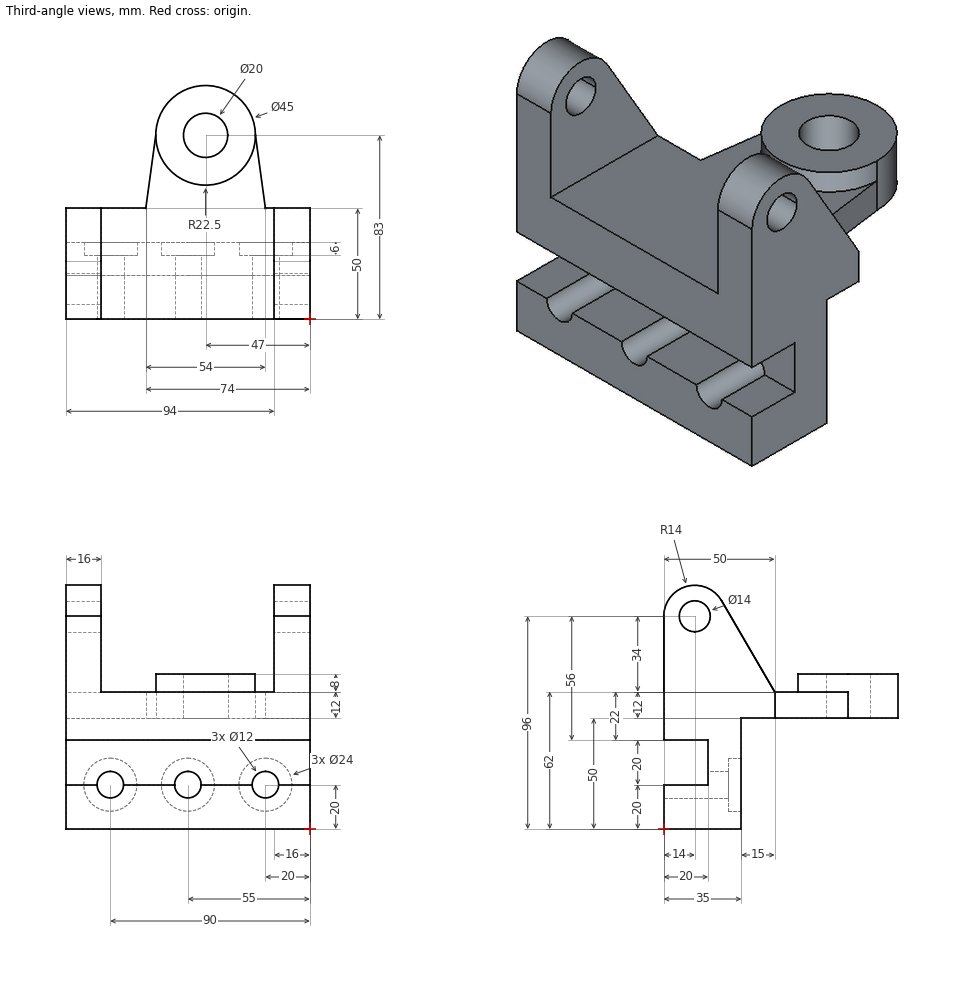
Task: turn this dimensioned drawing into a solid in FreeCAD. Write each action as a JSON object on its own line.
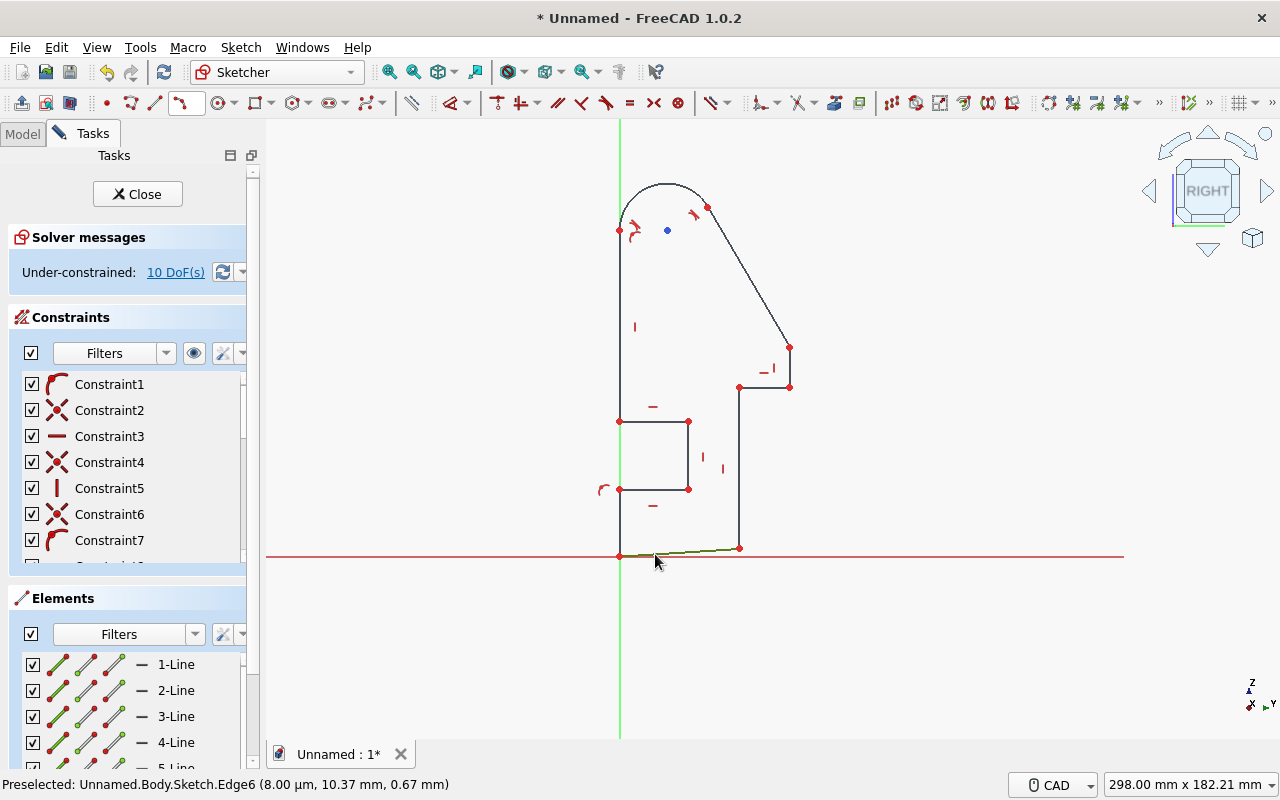
{"action": "left_click", "coordinate": [540, 104]}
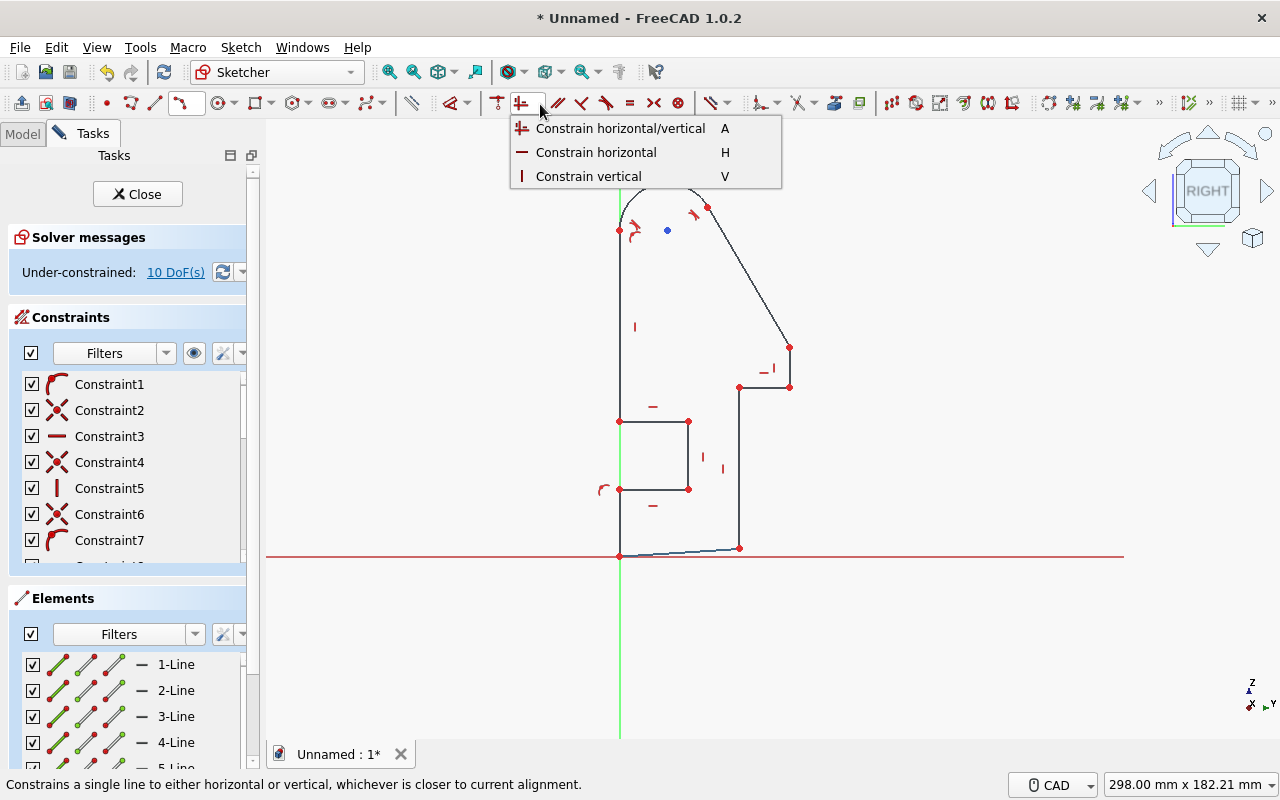
{"action": "left_click", "coordinate": [646, 152]}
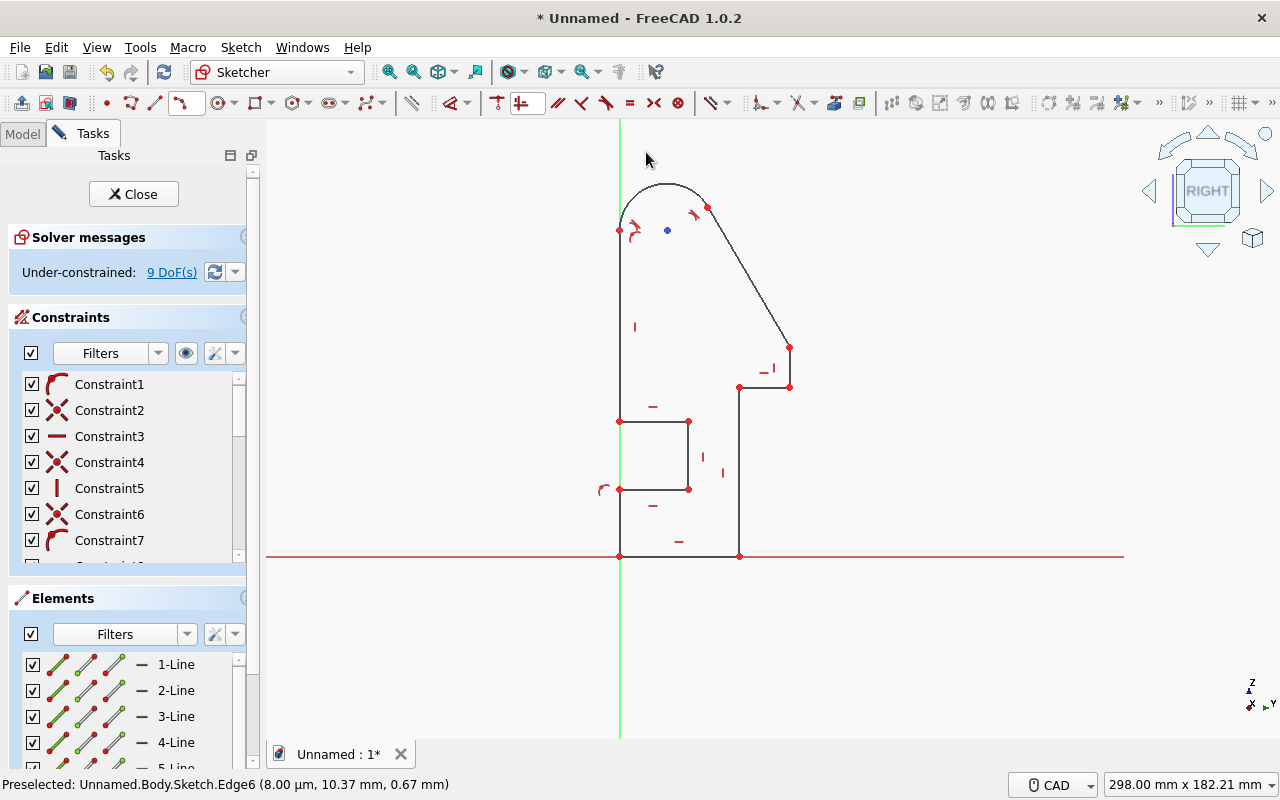
{"action": "left_click", "coordinate": [450, 104]}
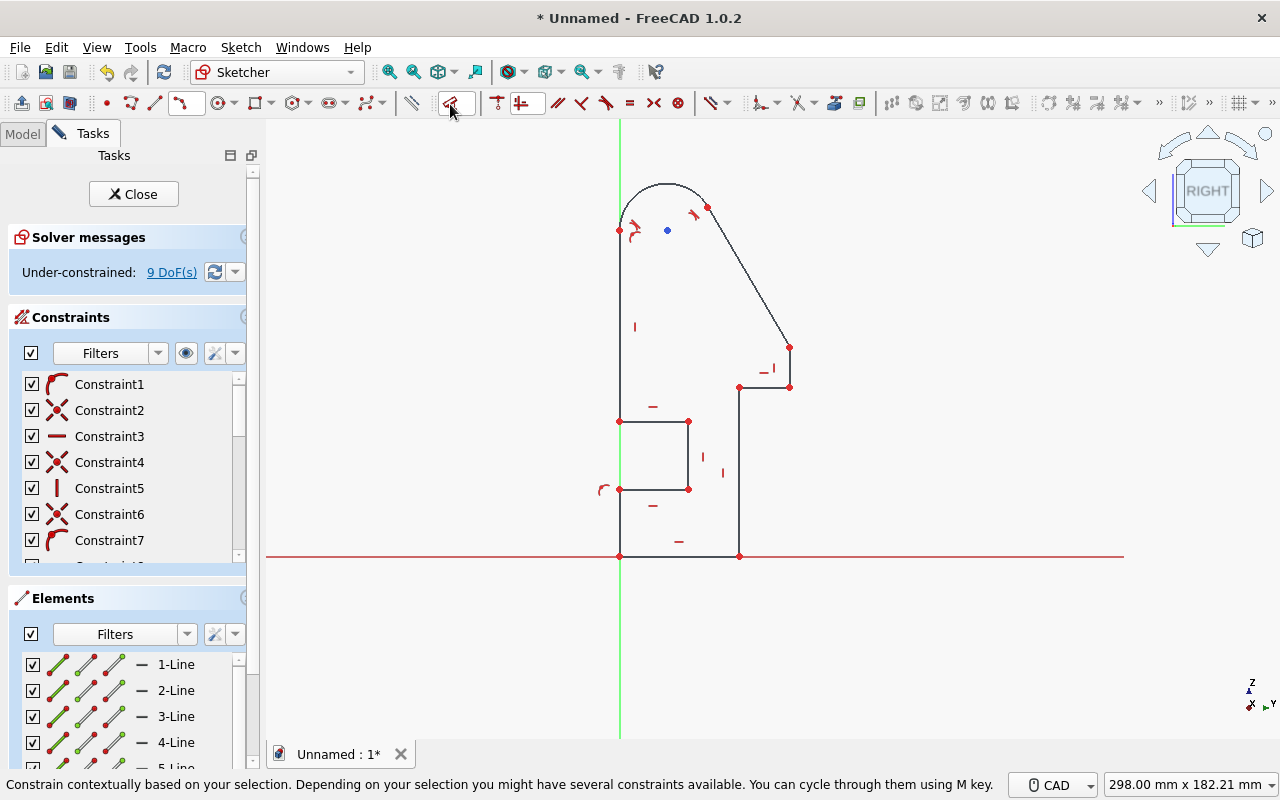
{"action": "left_click", "coordinate": [679, 185]}
{"action": "left_click", "coordinate": [687, 154]}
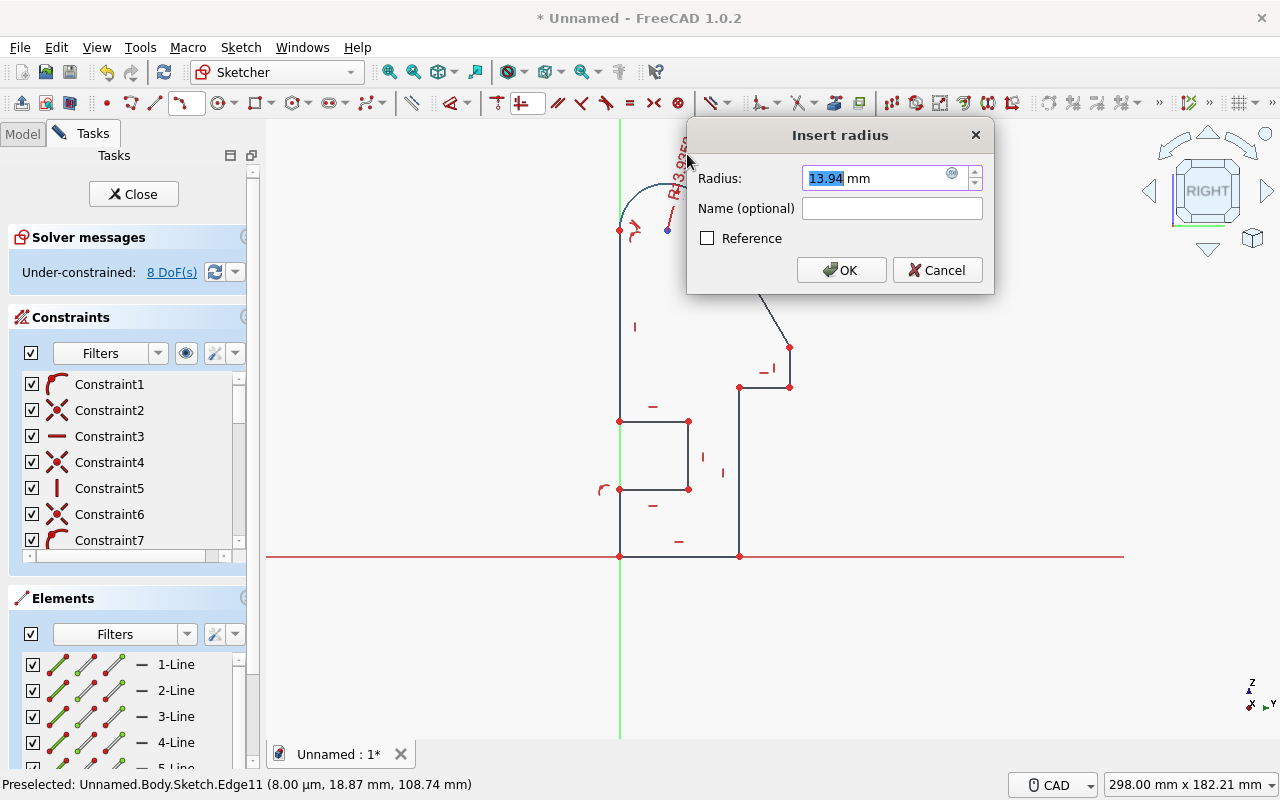
{"action": "type", "text": "14"}
{"action": "key", "text": "Return"}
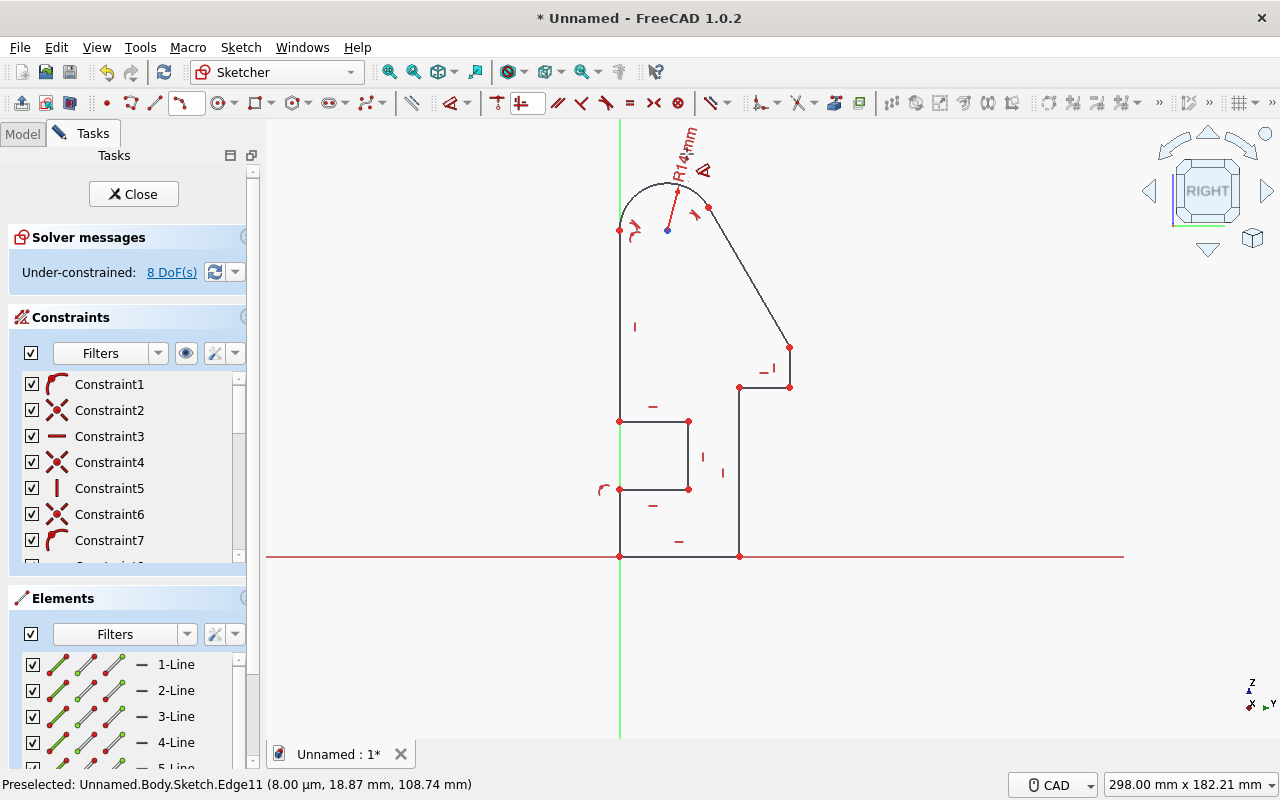
{"action": "left_click", "coordinate": [620, 288]}
{"action": "left_click", "coordinate": [586, 326]}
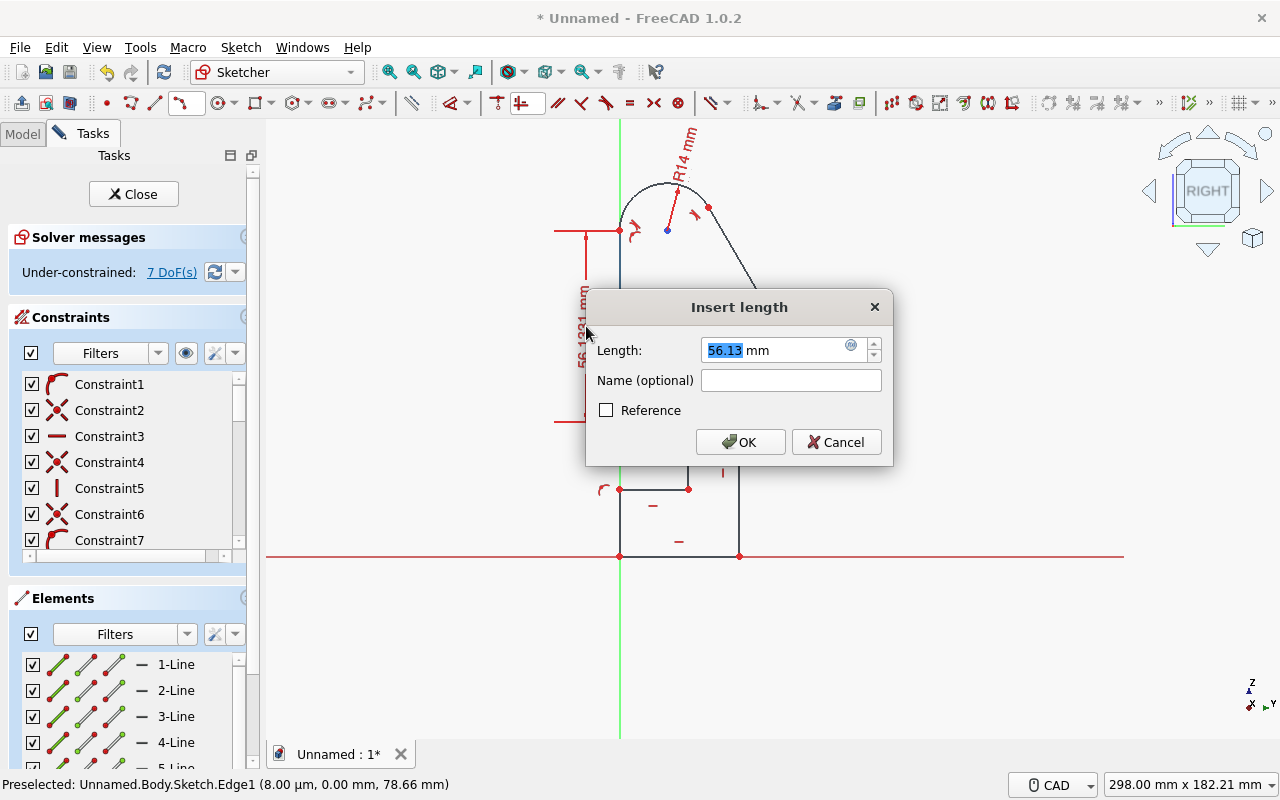
{"action": "type", "text": "56"}
{"action": "key", "text": "Return"}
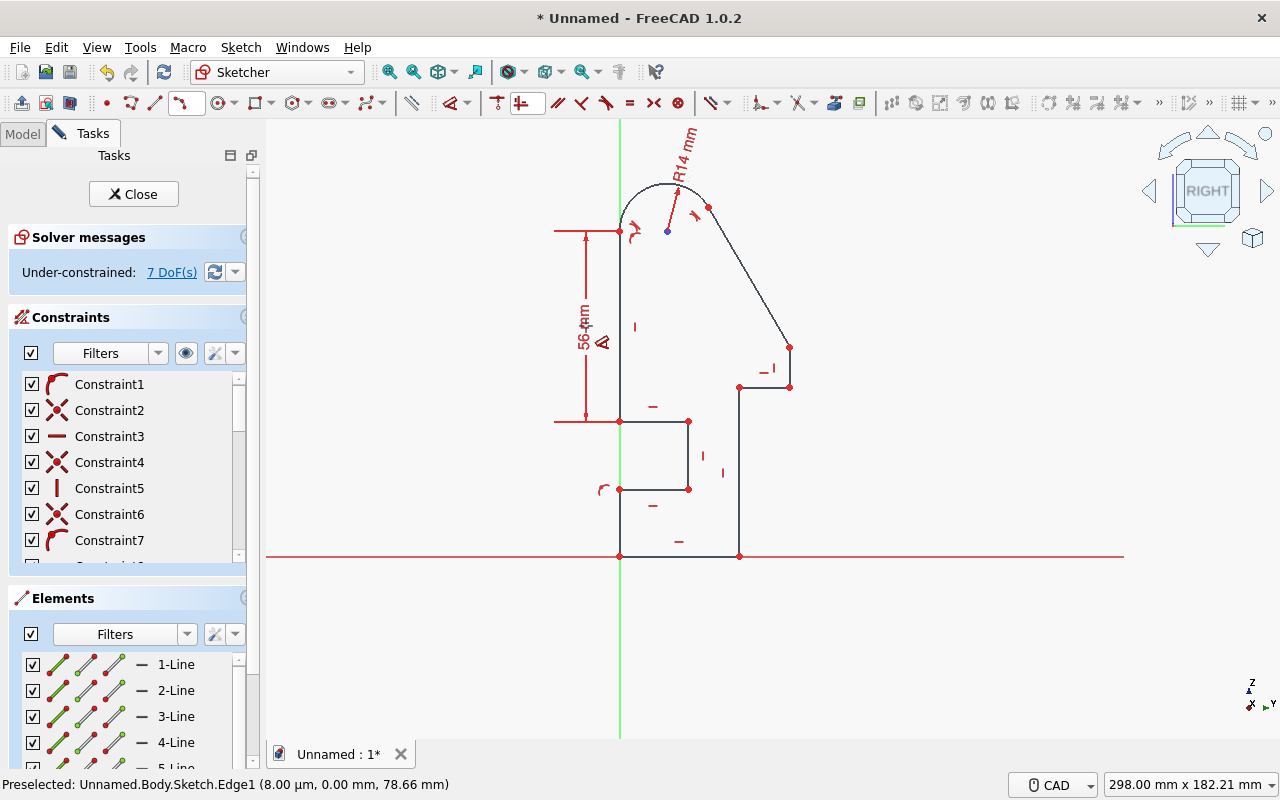
{"action": "left_click", "coordinate": [640, 422]}
{"action": "left_click", "coordinate": [654, 456]}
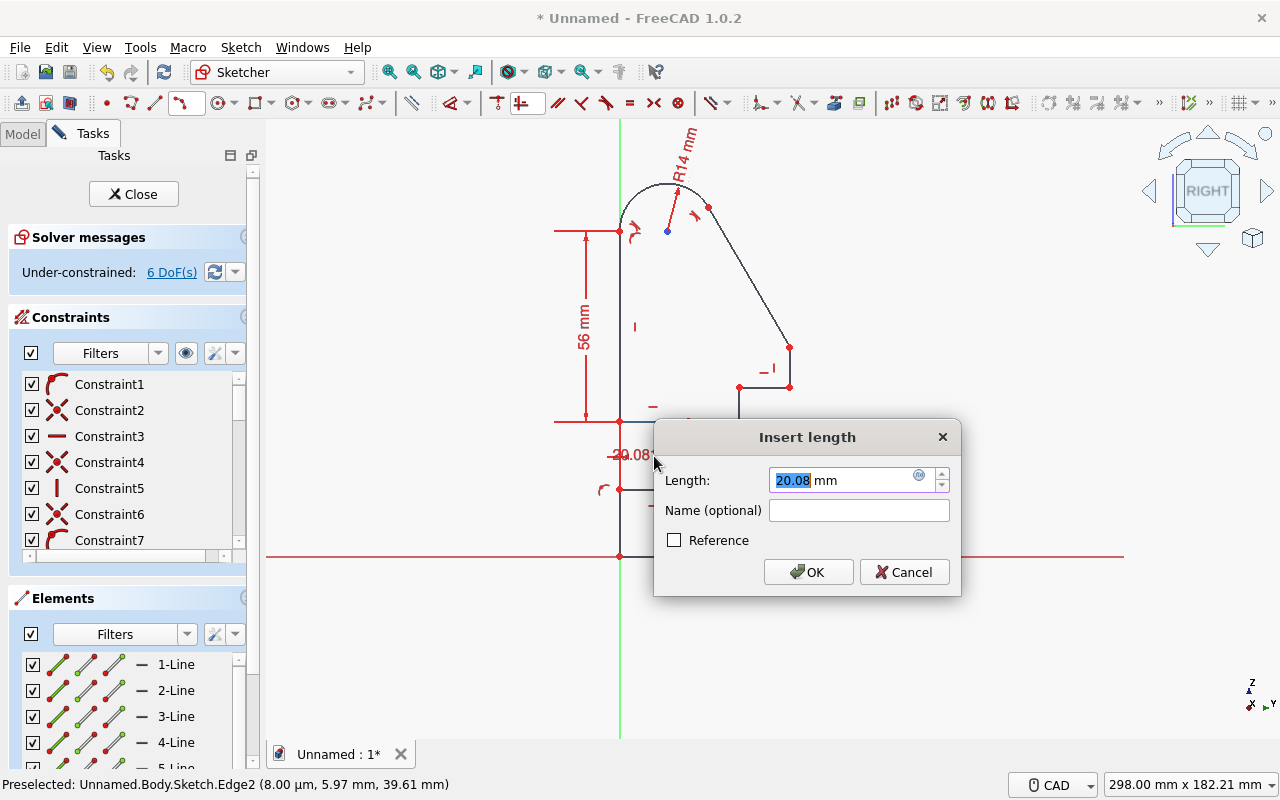
{"action": "type", "text": "20"}
{"action": "key", "text": "Return"}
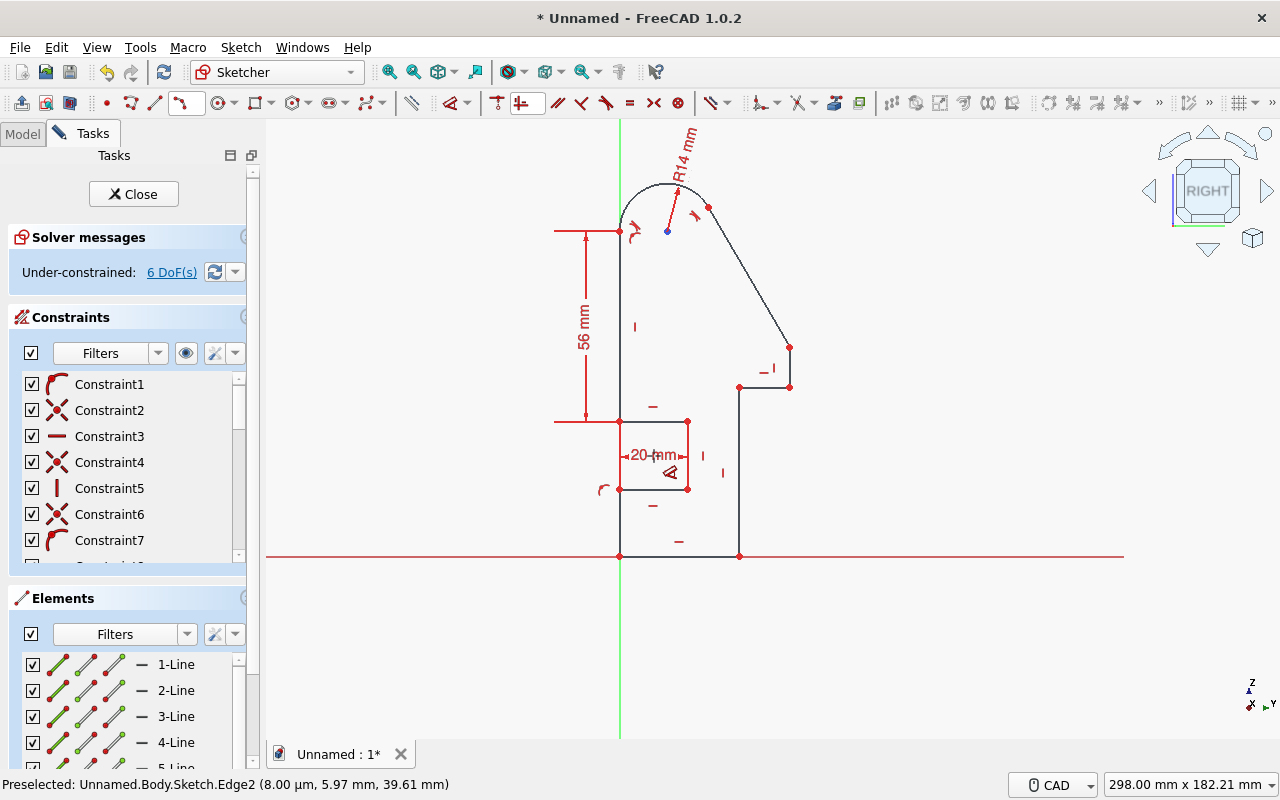
{"action": "left_click", "coordinate": [688, 442]}
{"action": "left_click", "coordinate": [722, 432]}